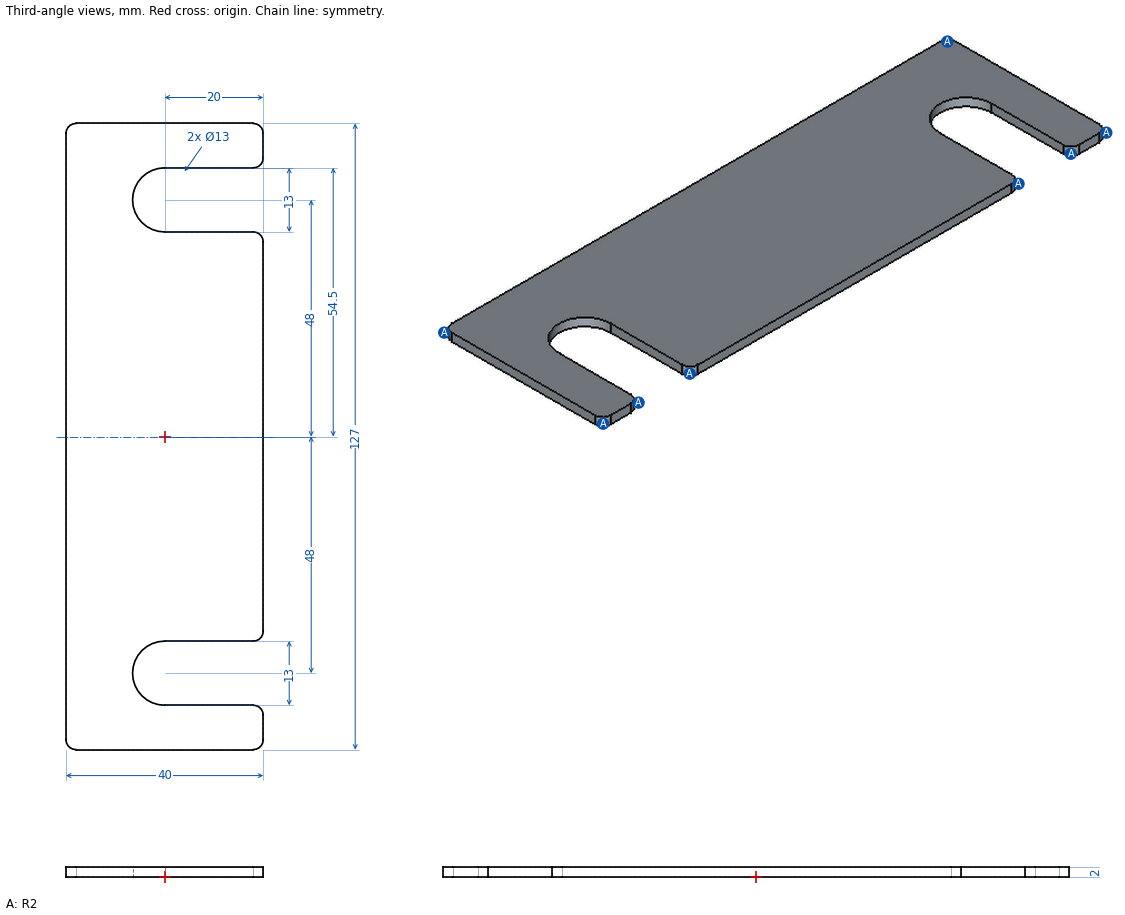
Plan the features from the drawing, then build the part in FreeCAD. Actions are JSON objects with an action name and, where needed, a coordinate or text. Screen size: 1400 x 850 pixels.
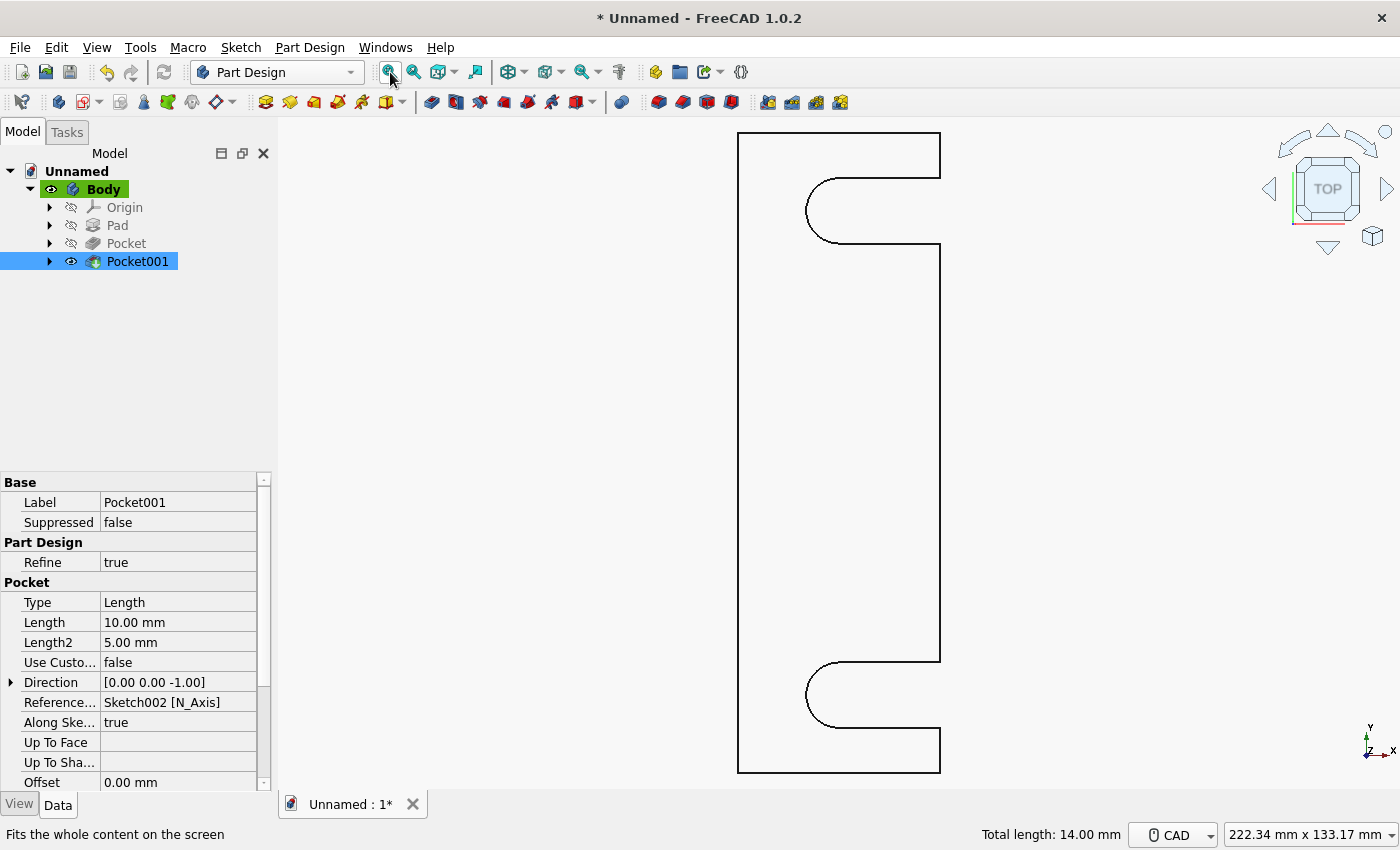
{"action": "key", "text": "1"}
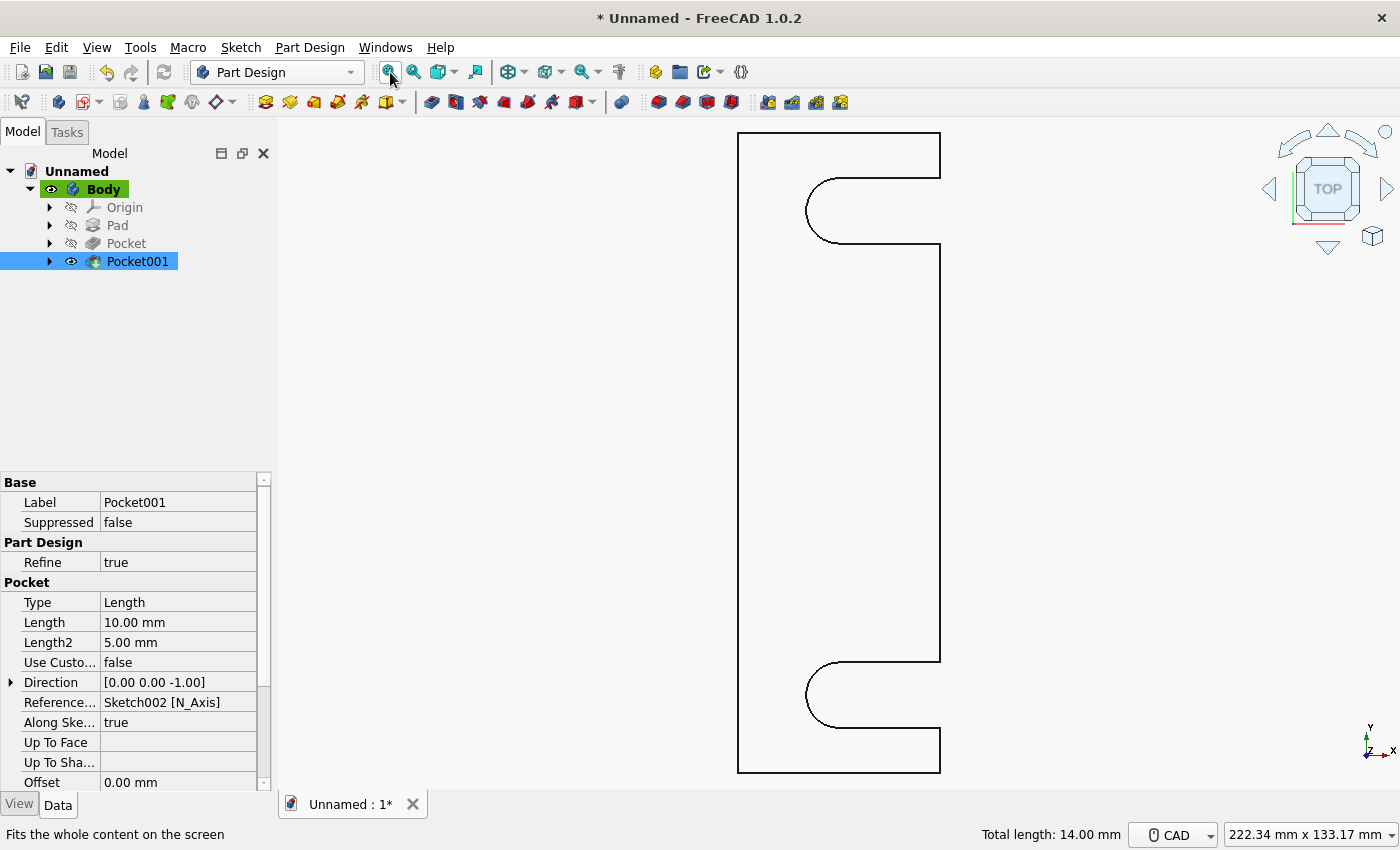
{"action": "left_click", "coordinate": [390, 72]}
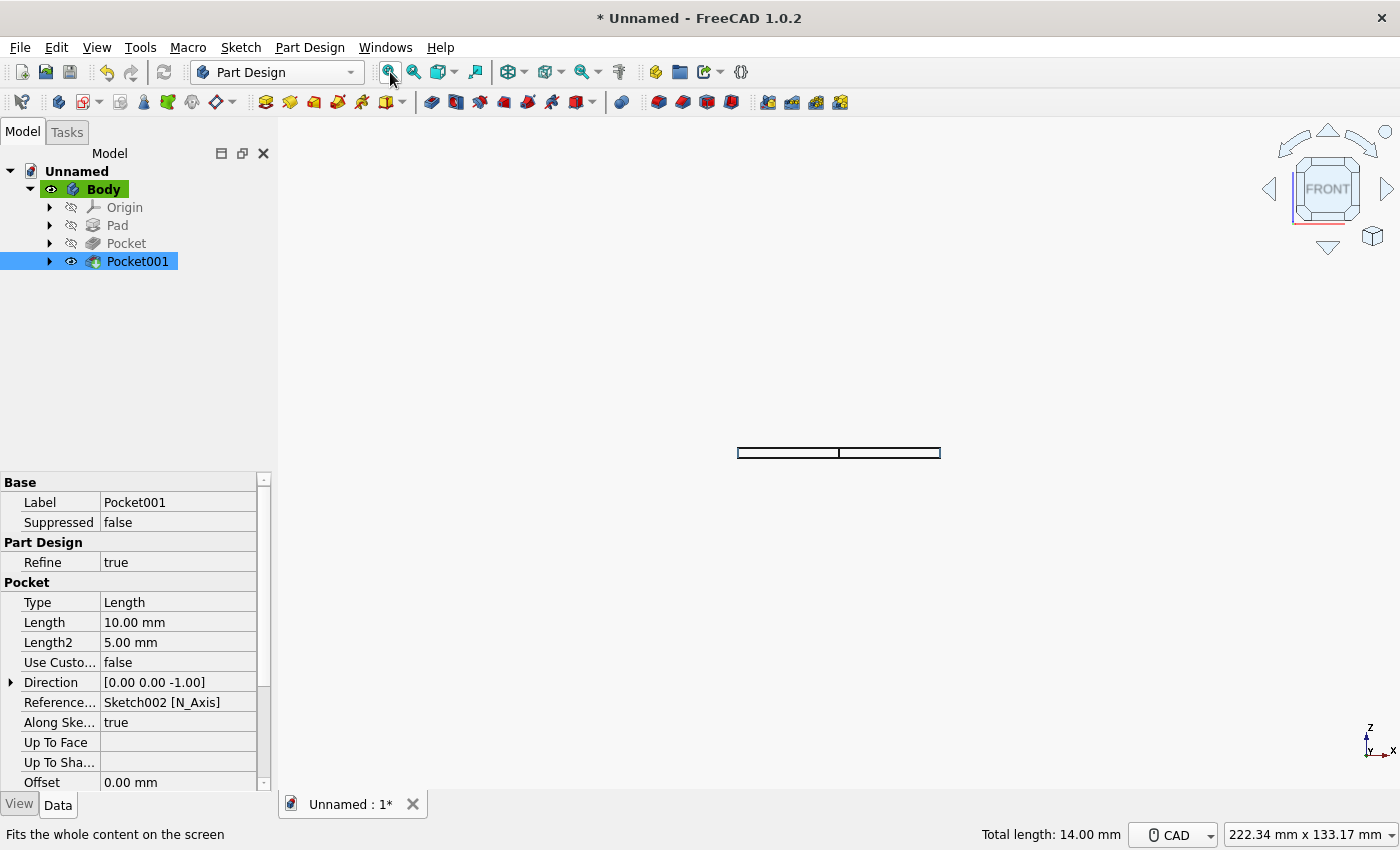
{"action": "scroll", "coordinate": [738, 452], "scroll_direction": "up", "scroll_amount": 7}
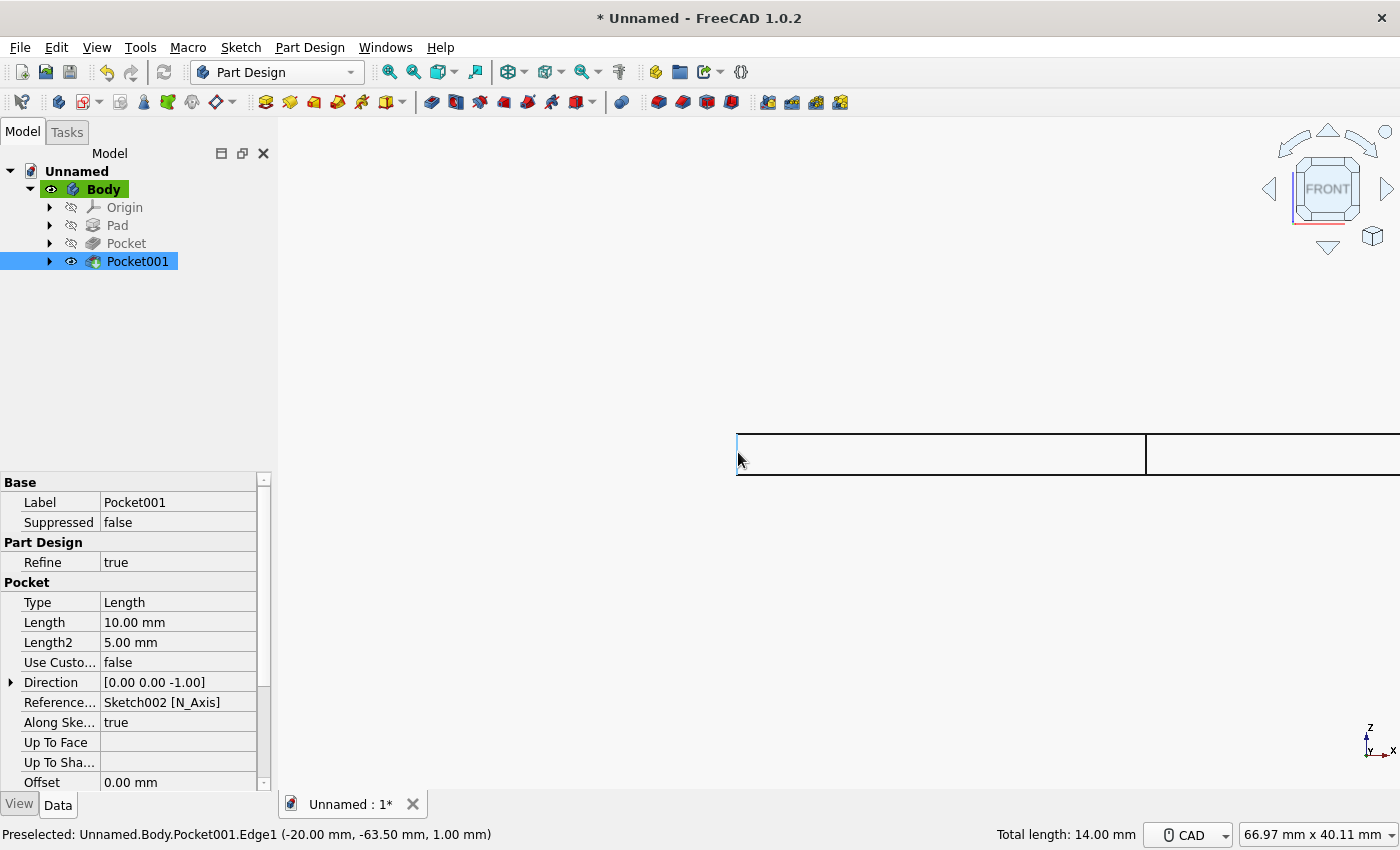
{"action": "left_click", "coordinate": [390, 72]}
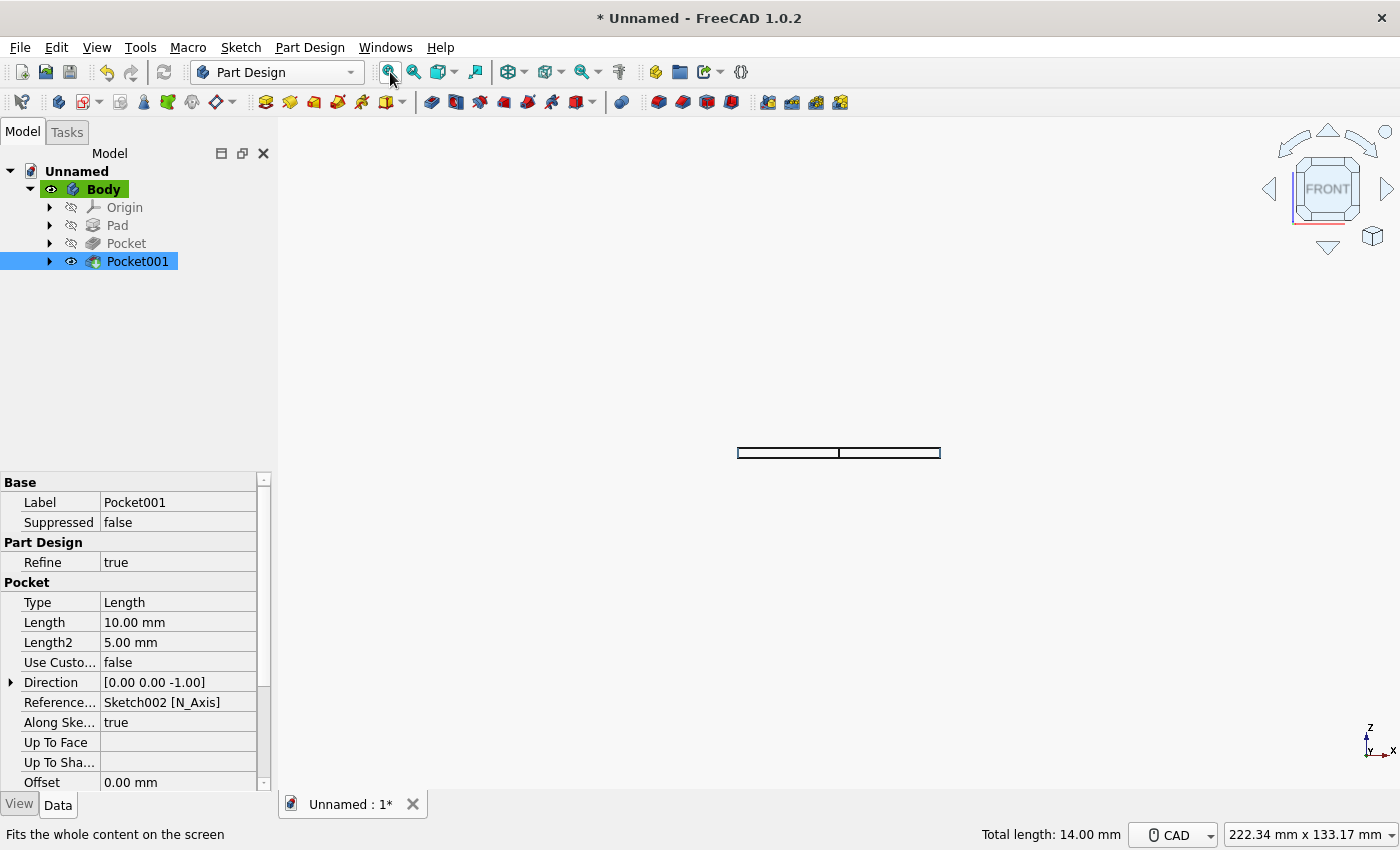
{"action": "key", "text": "3"}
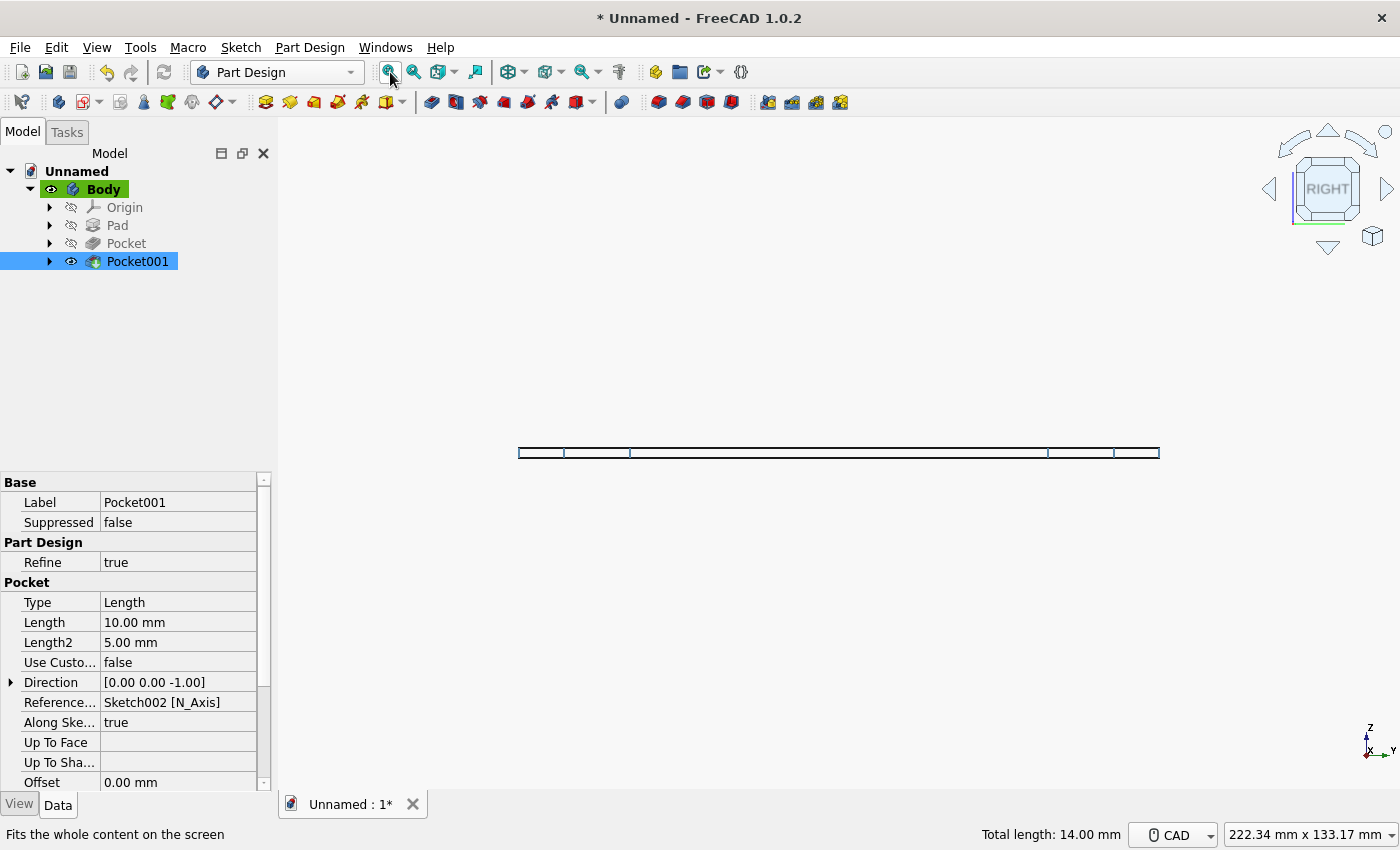
{"action": "scroll", "coordinate": [1159, 452], "scroll_direction": "up", "scroll_amount": 7}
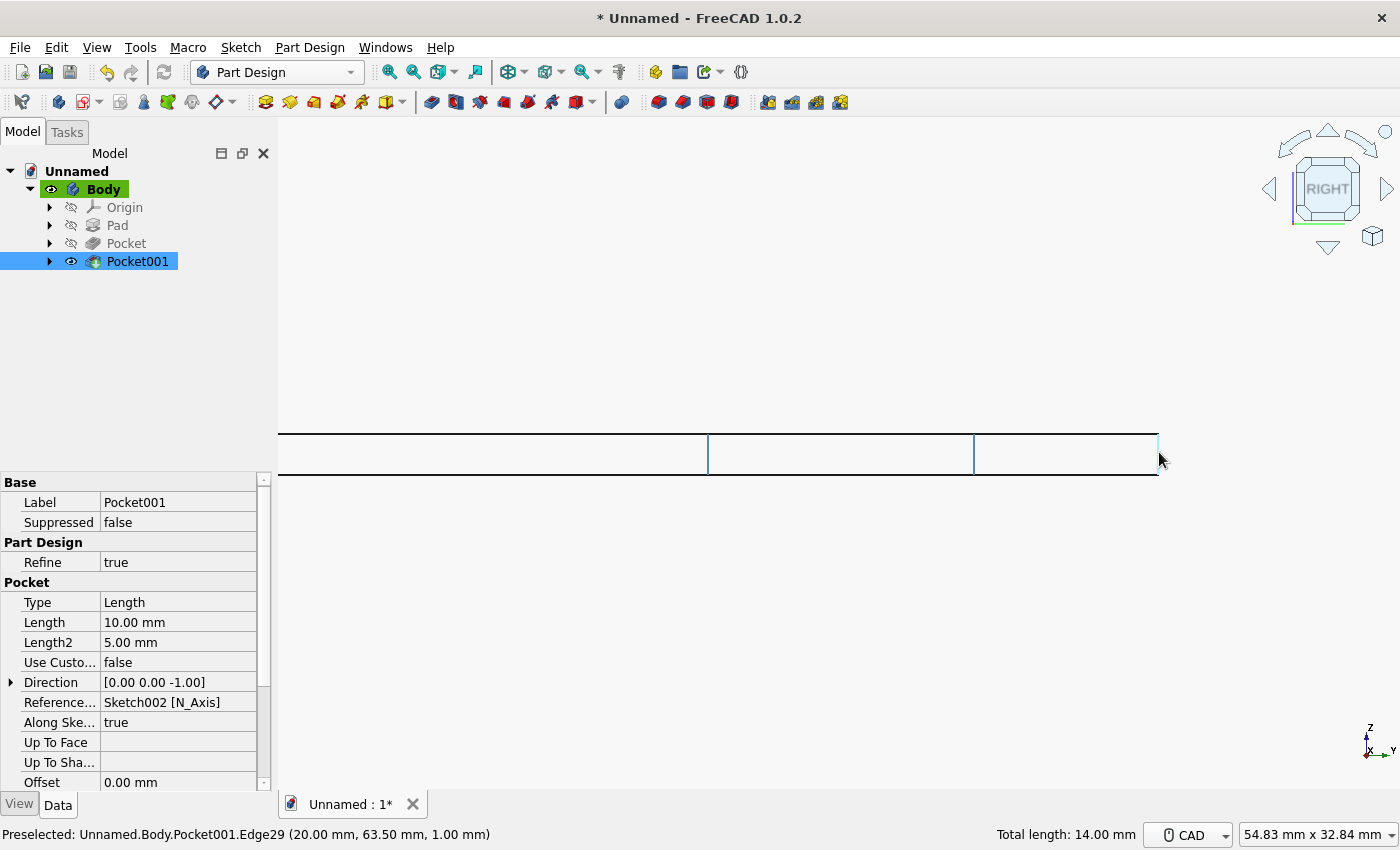
{"action": "left_click", "coordinate": [390, 72]}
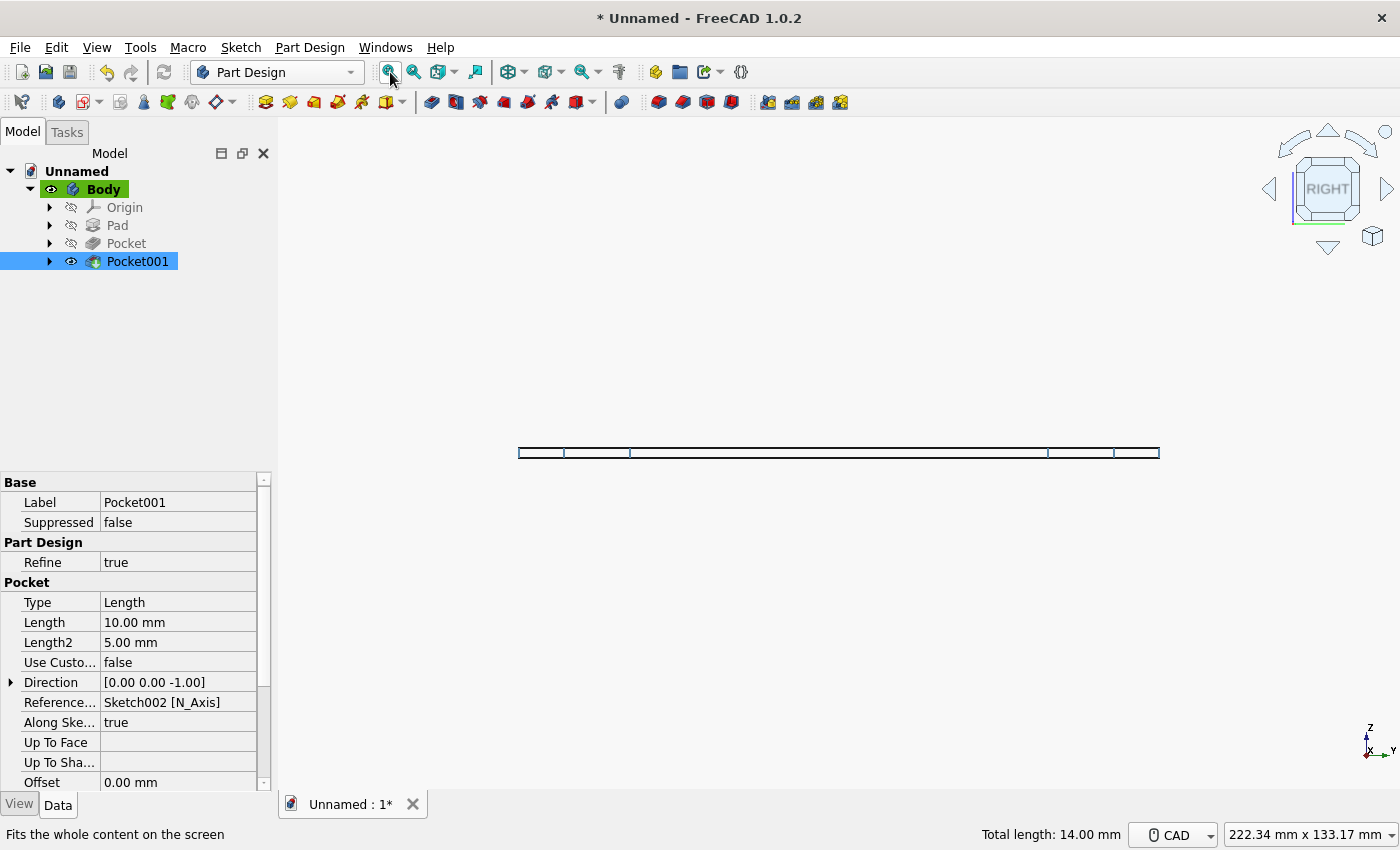
{"action": "key", "text": "5"}